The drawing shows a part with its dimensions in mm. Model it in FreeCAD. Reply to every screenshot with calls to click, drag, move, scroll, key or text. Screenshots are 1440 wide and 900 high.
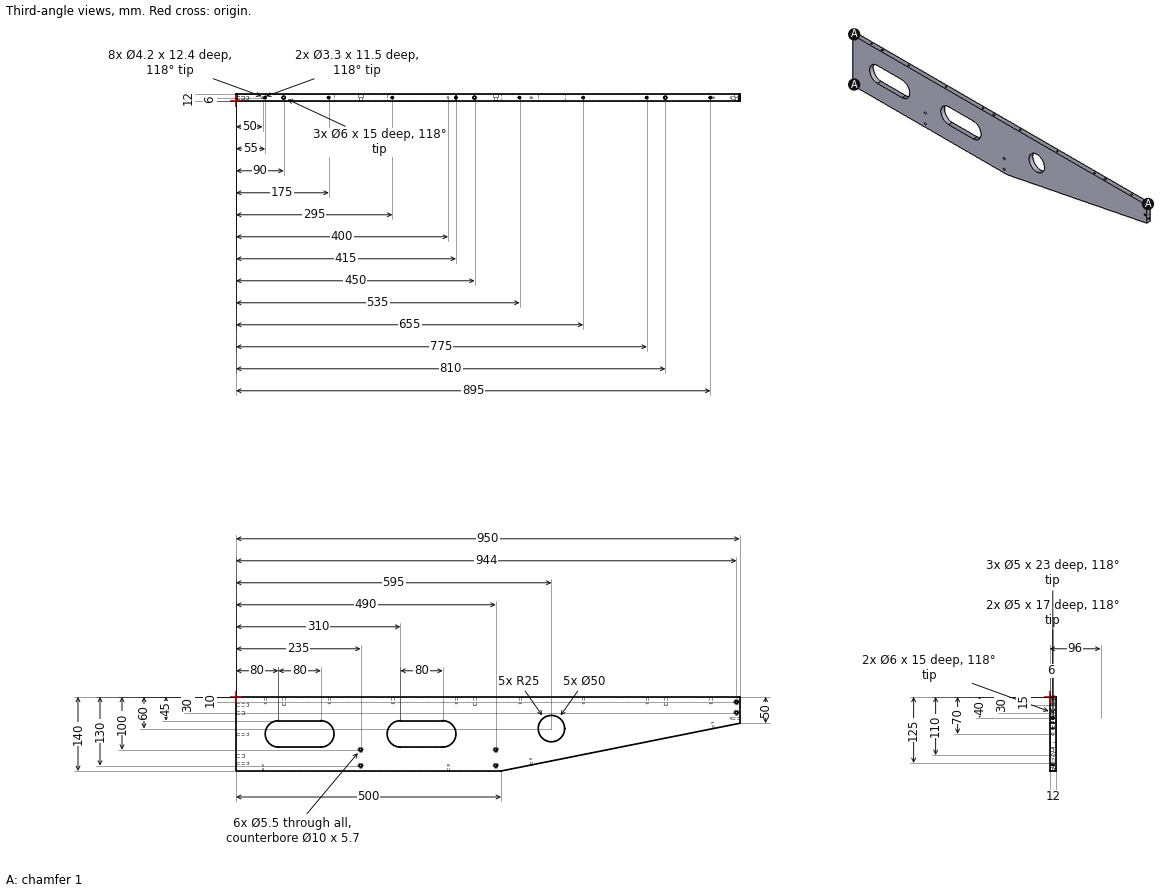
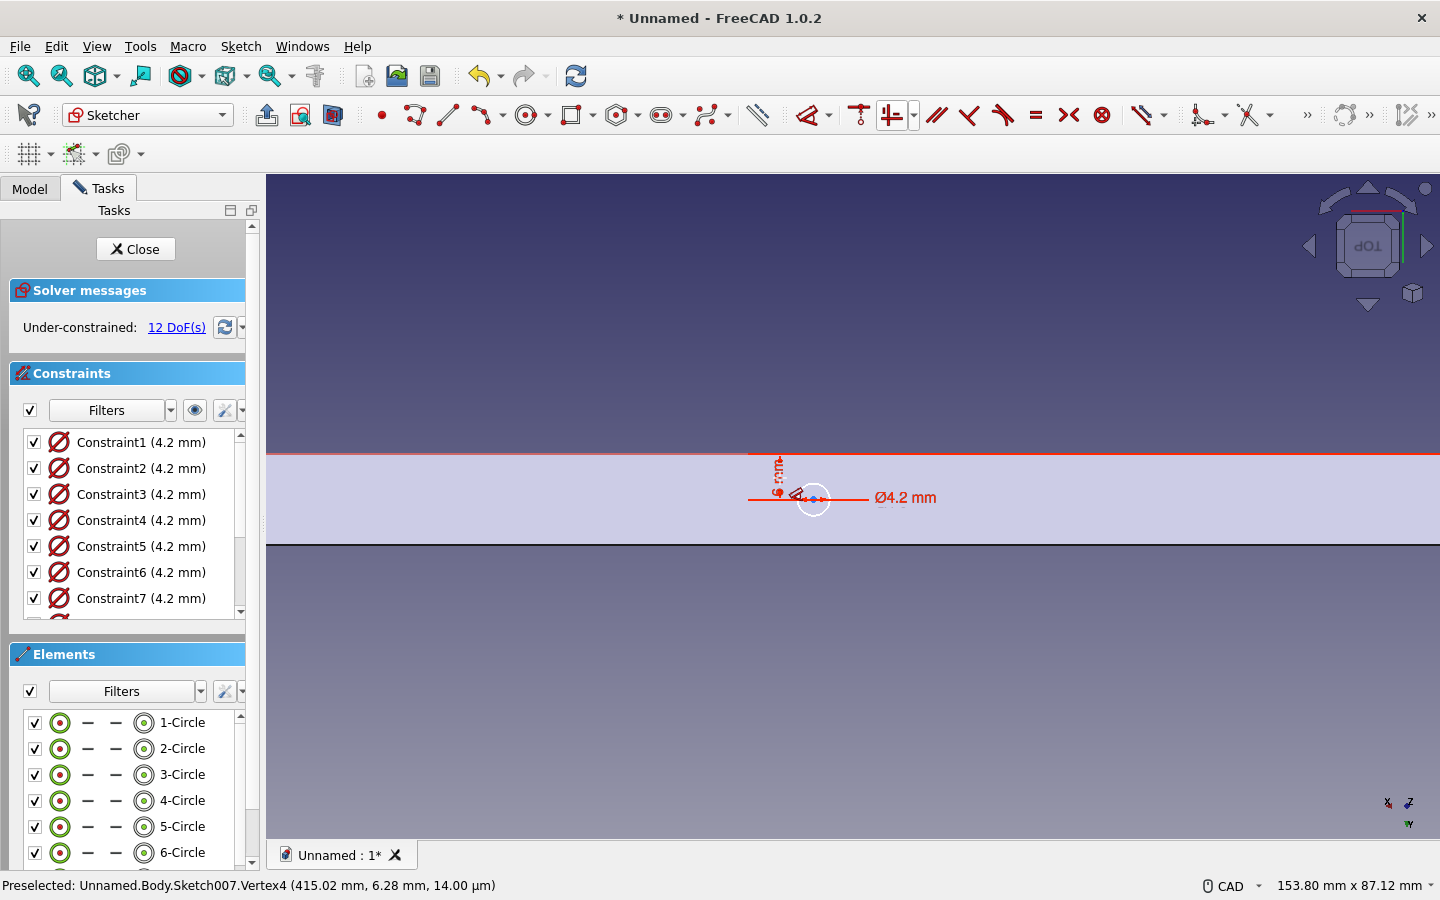
scroll(813, 509, down, 11)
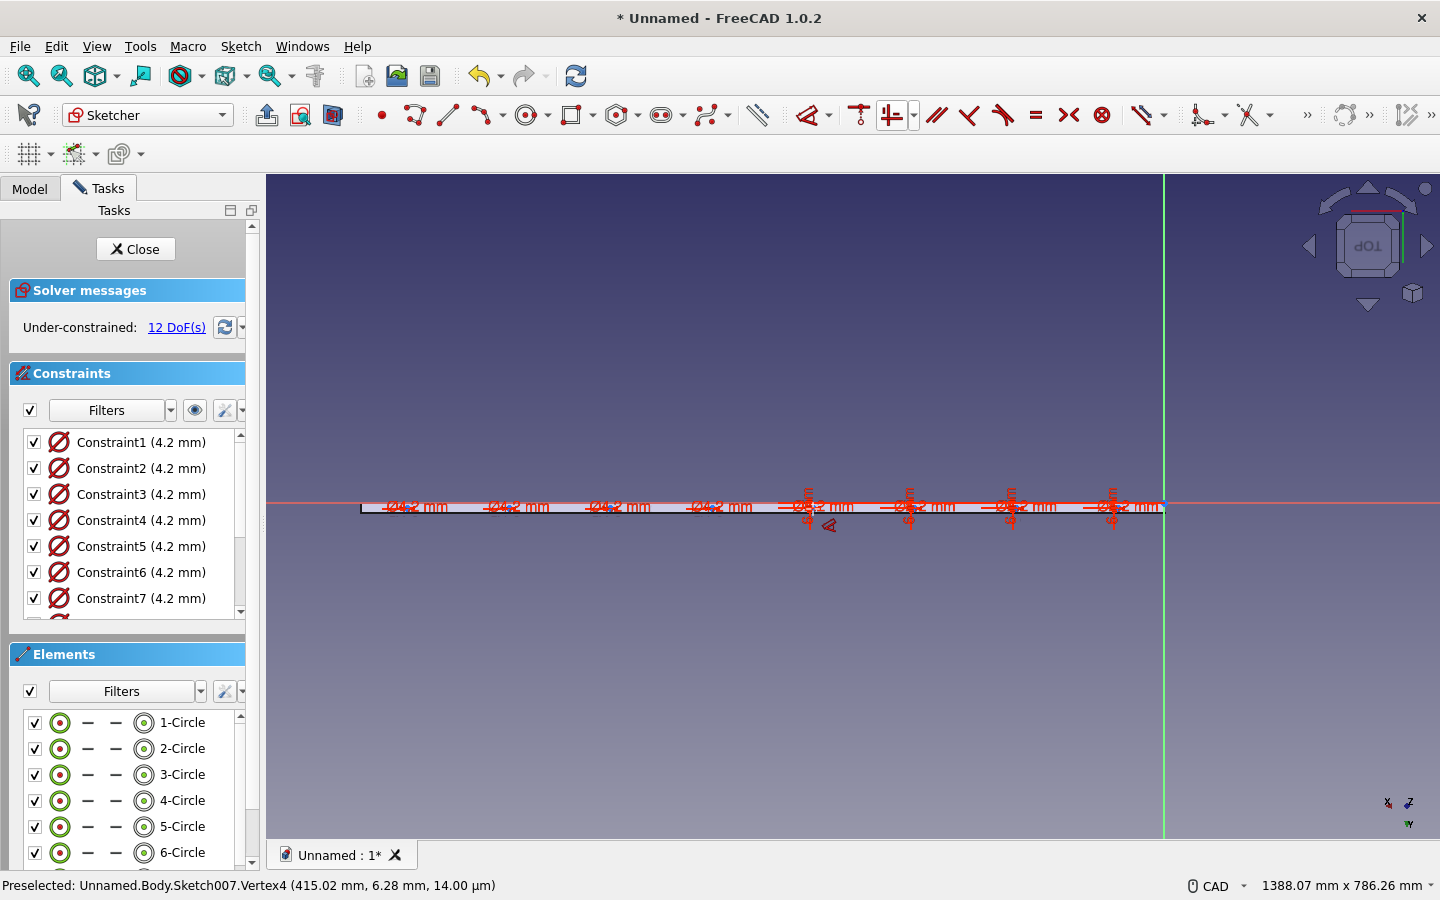
scroll(712, 509, up, 11)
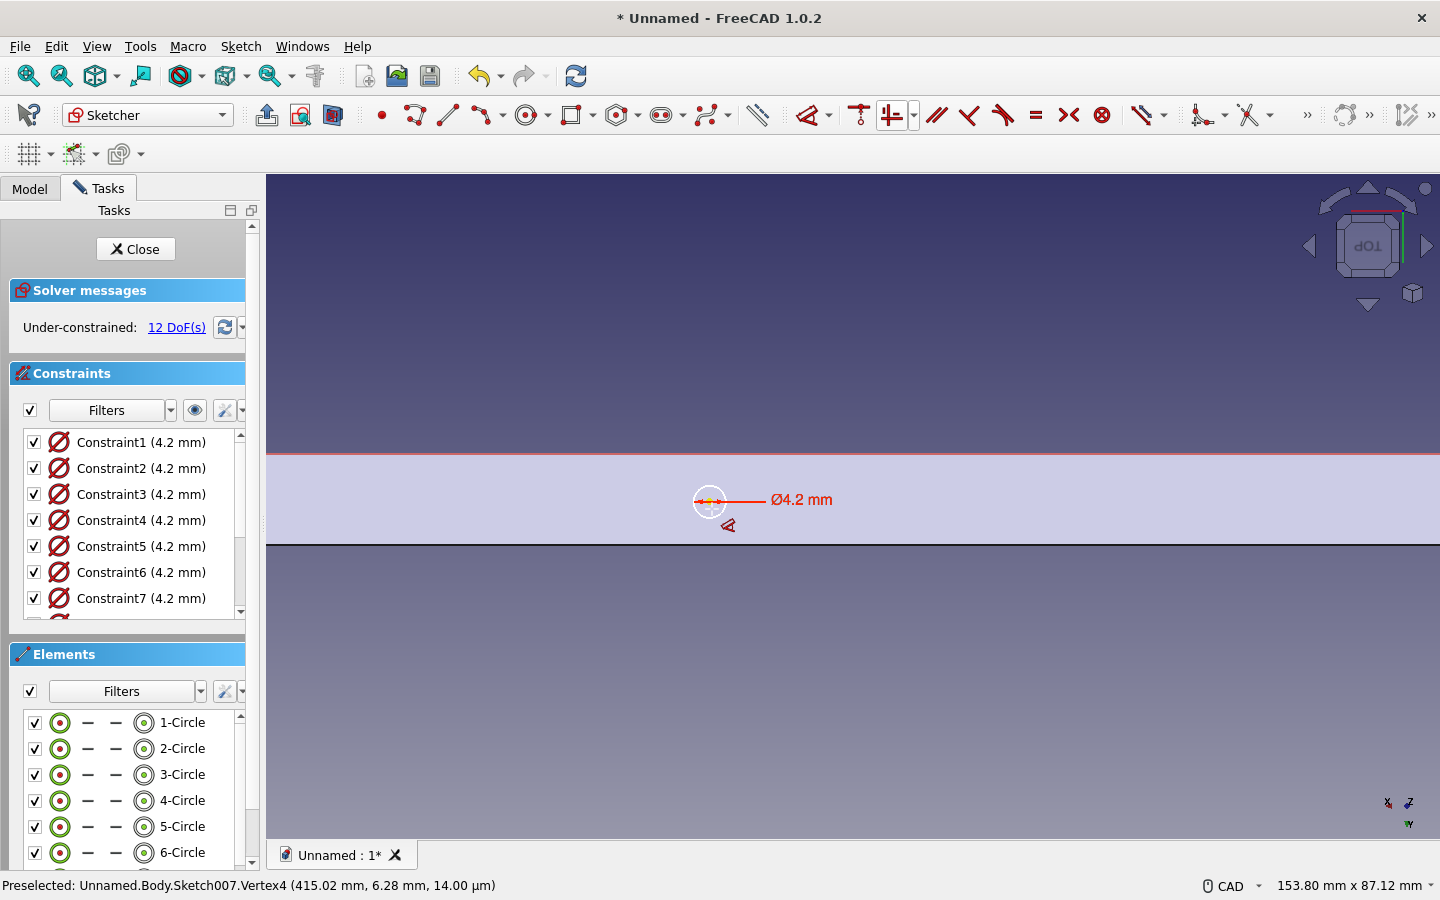
click(710, 502)
click(676, 478)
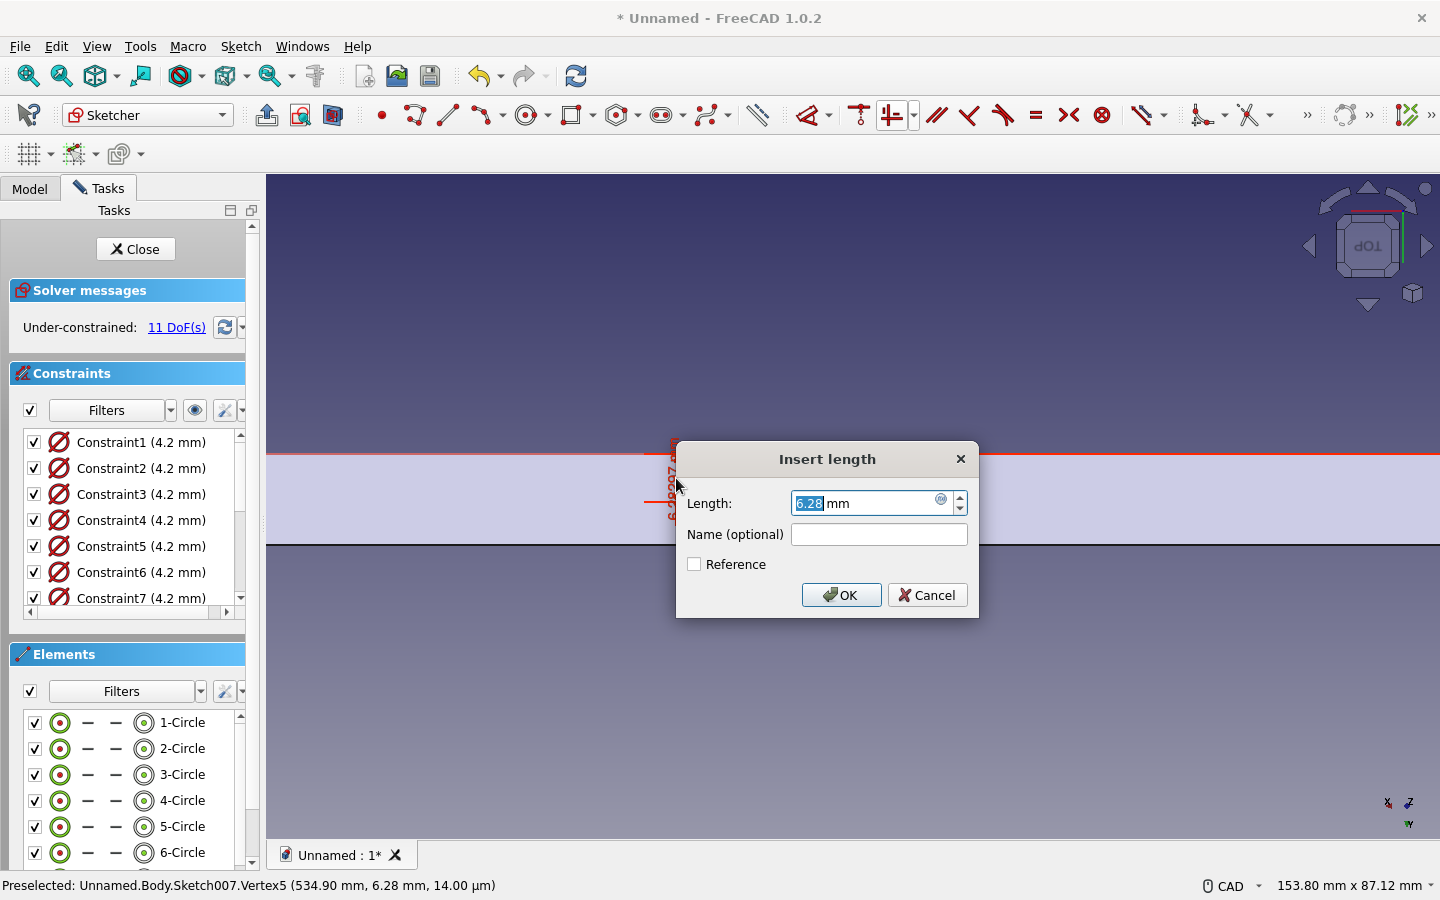
text(6)
key(Return)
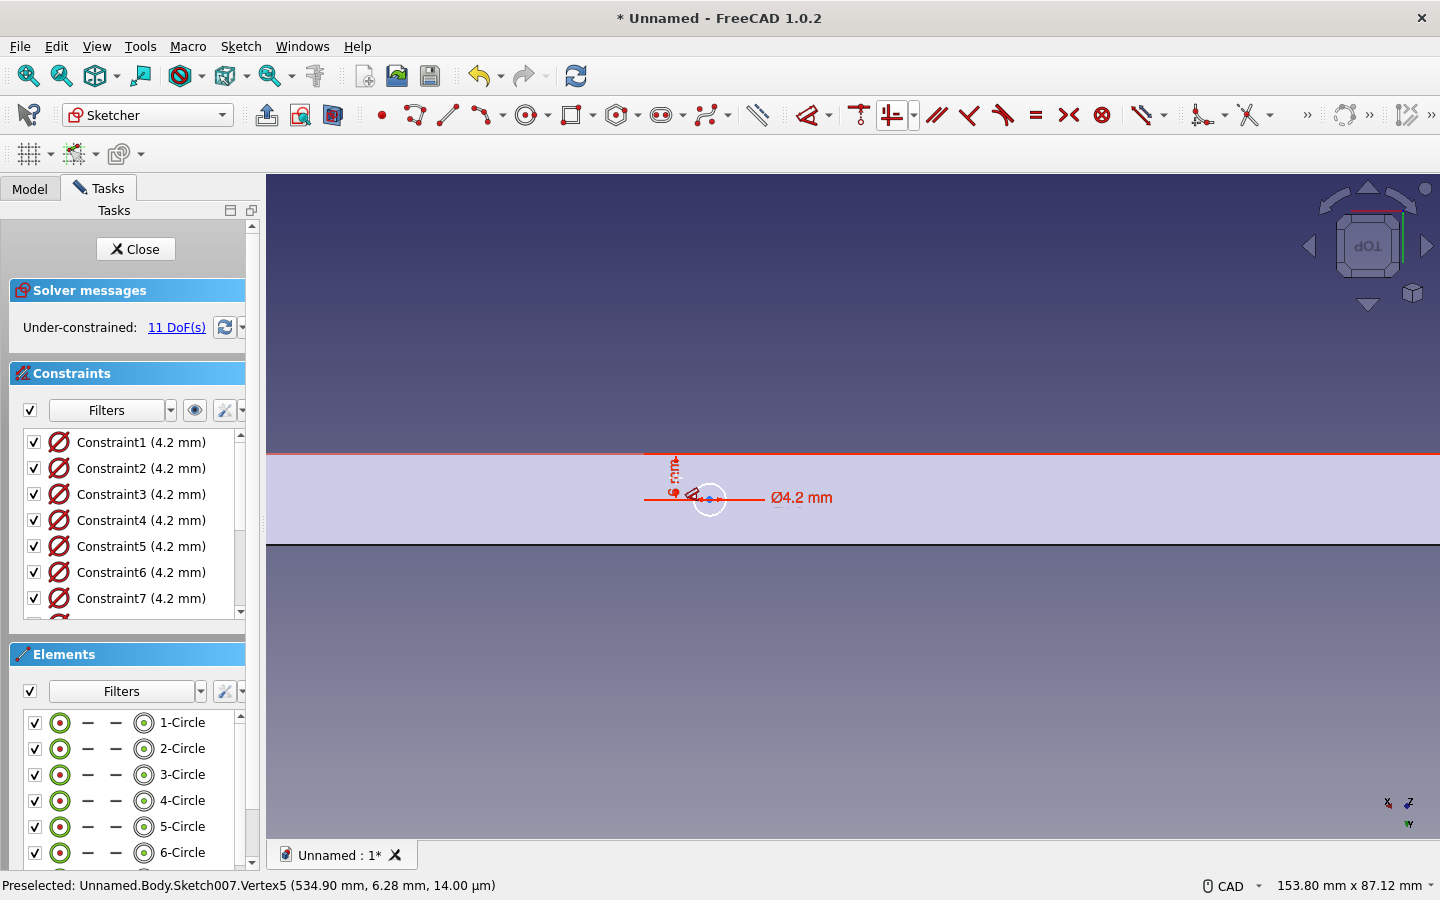
scroll(712, 509, down, 11)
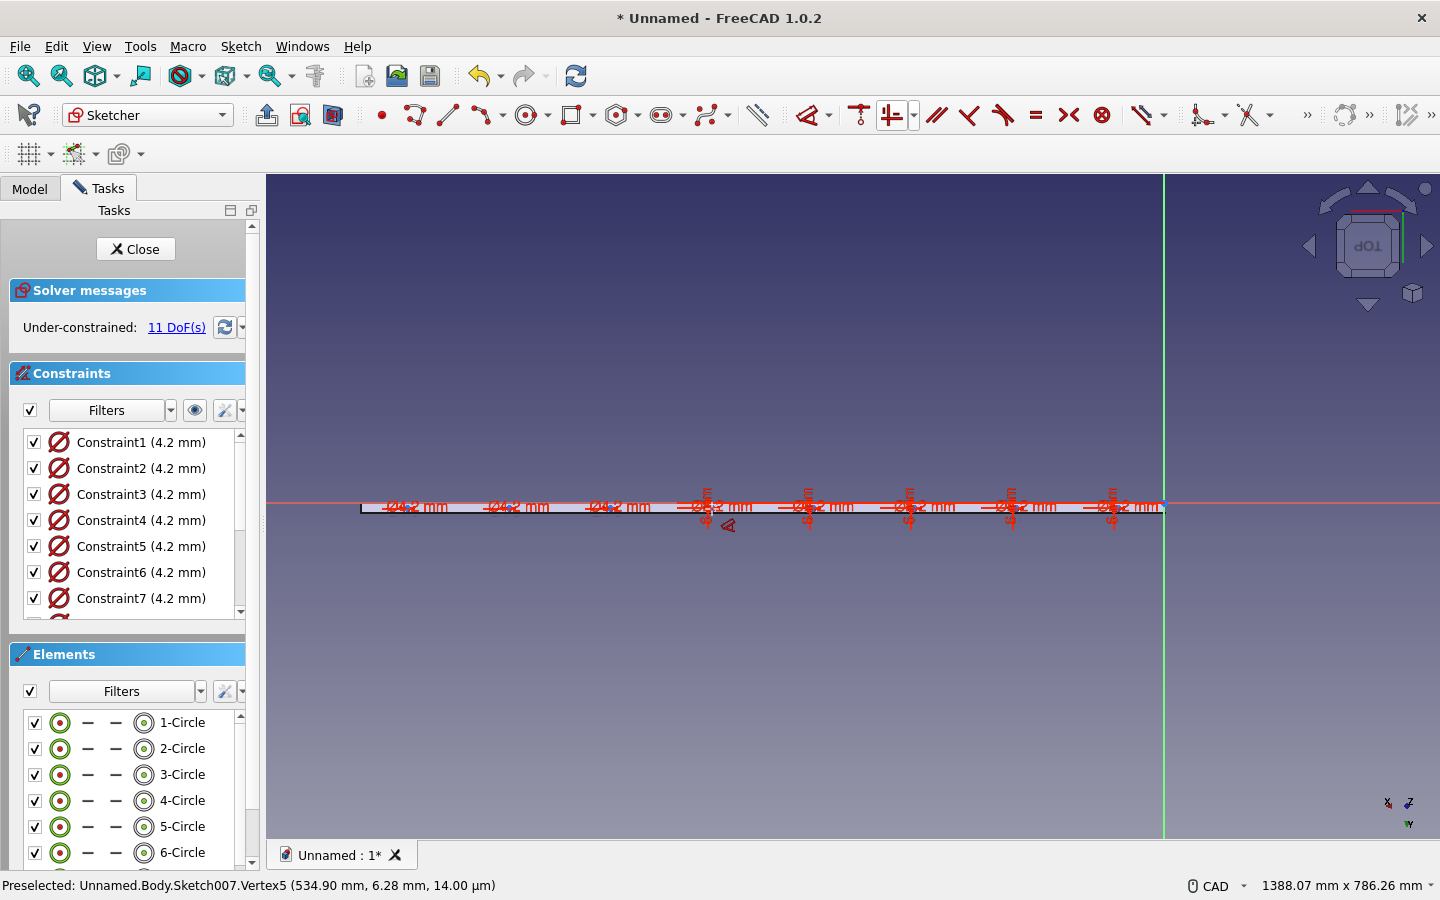
scroll(610, 509, up, 11)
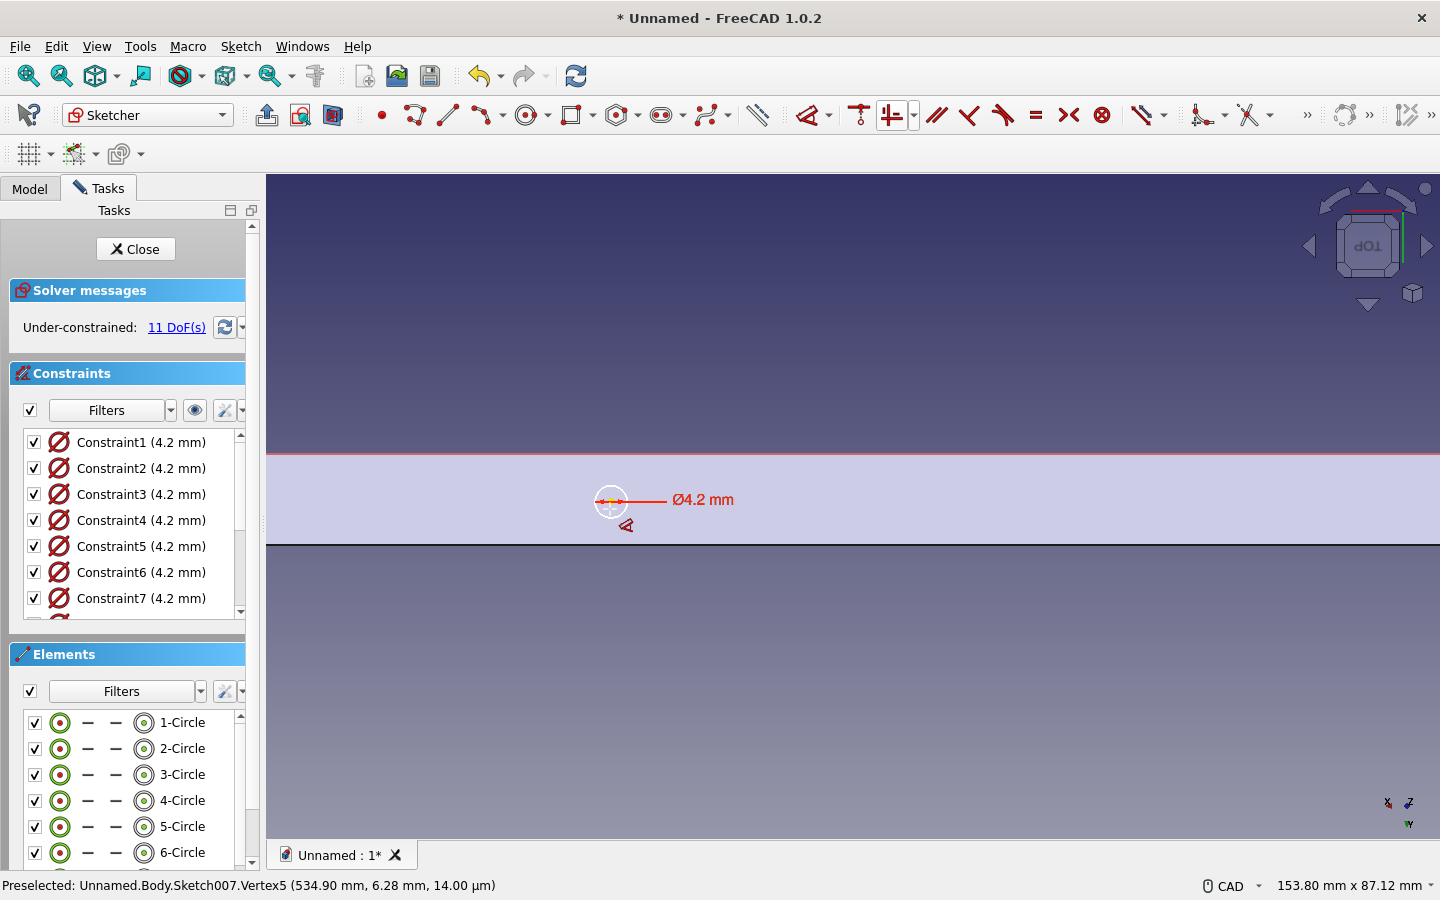
click(611, 502)
click(577, 478)